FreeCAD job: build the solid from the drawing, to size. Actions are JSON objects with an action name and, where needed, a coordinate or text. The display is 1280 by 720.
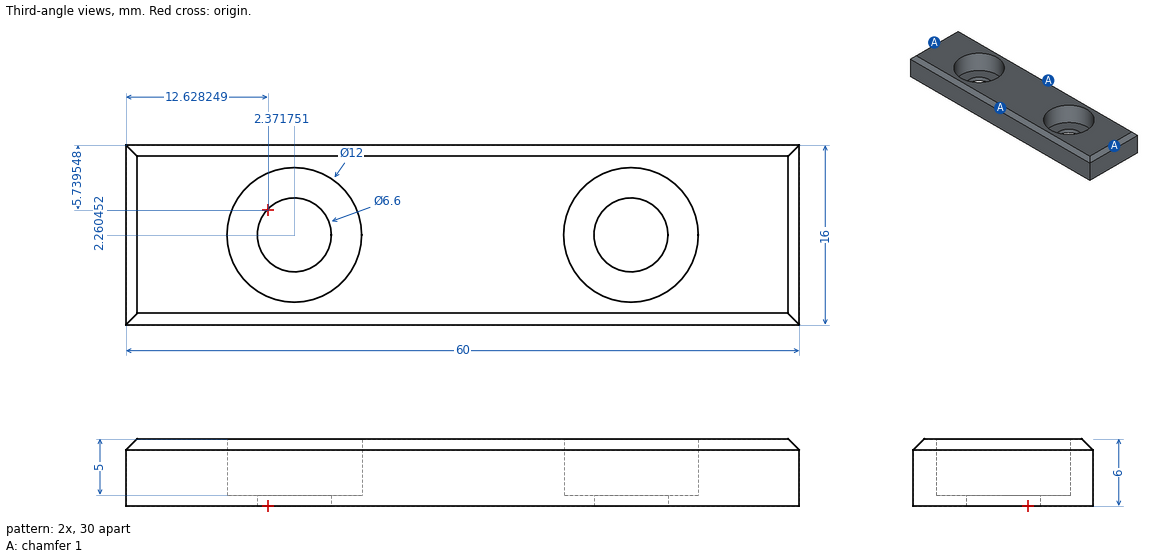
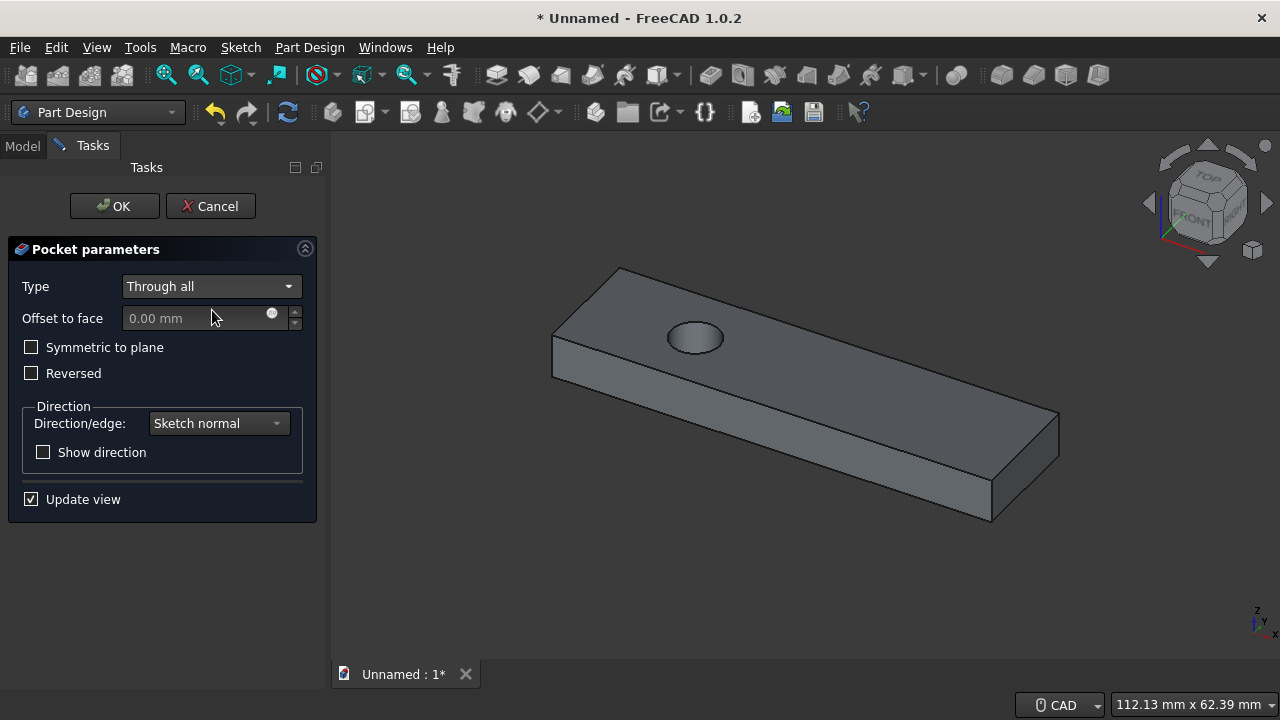
{"action": "left_click", "coordinate": [115, 206]}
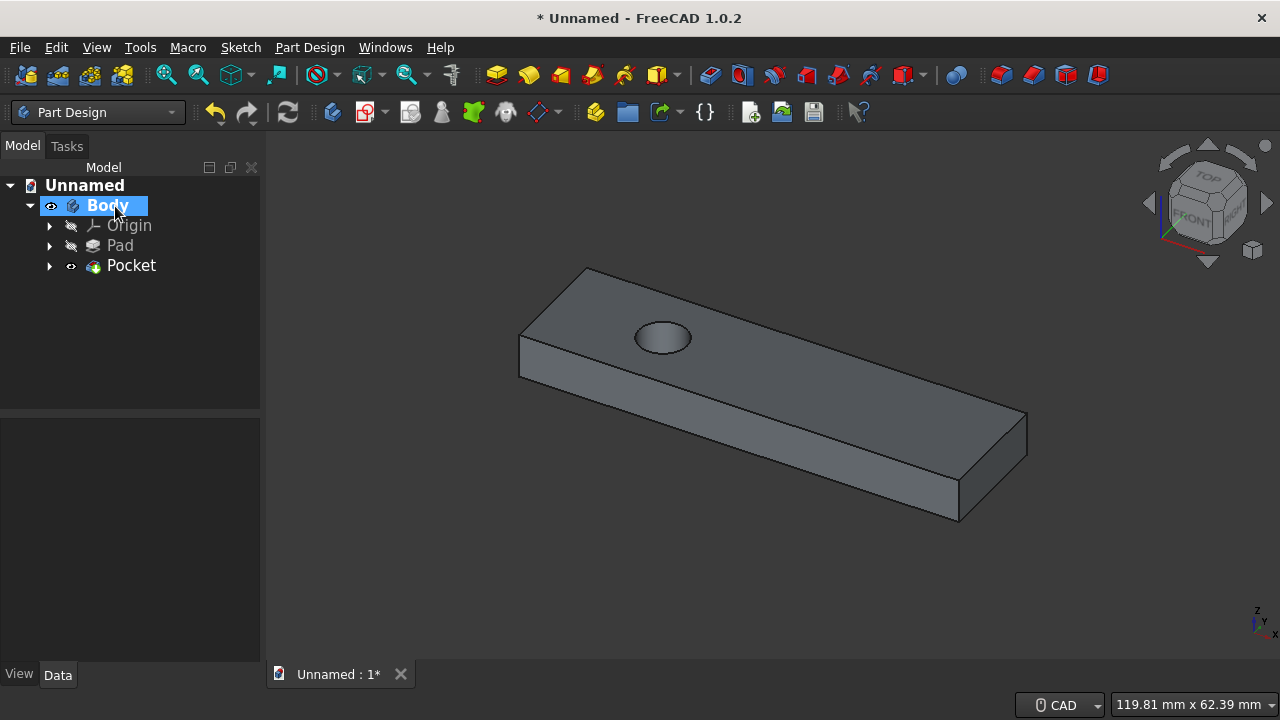
{"action": "left_click", "coordinate": [899, 415]}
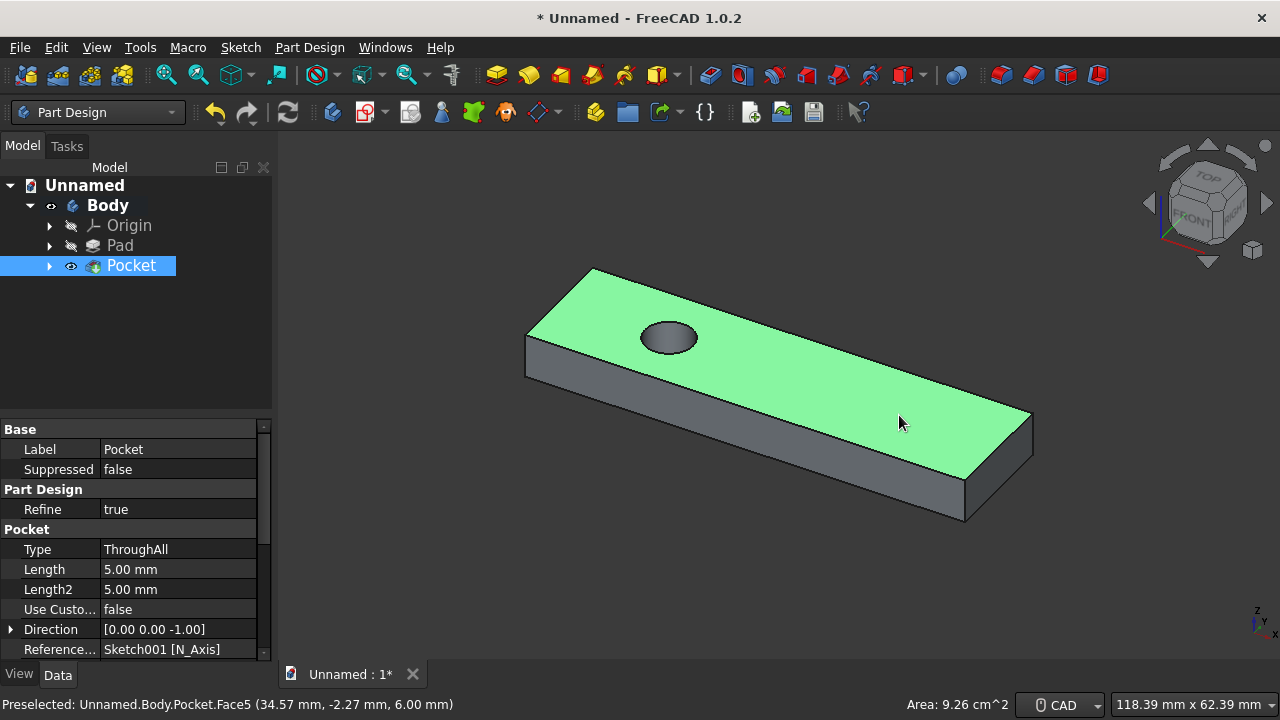
{"action": "left_click", "coordinate": [366, 112]}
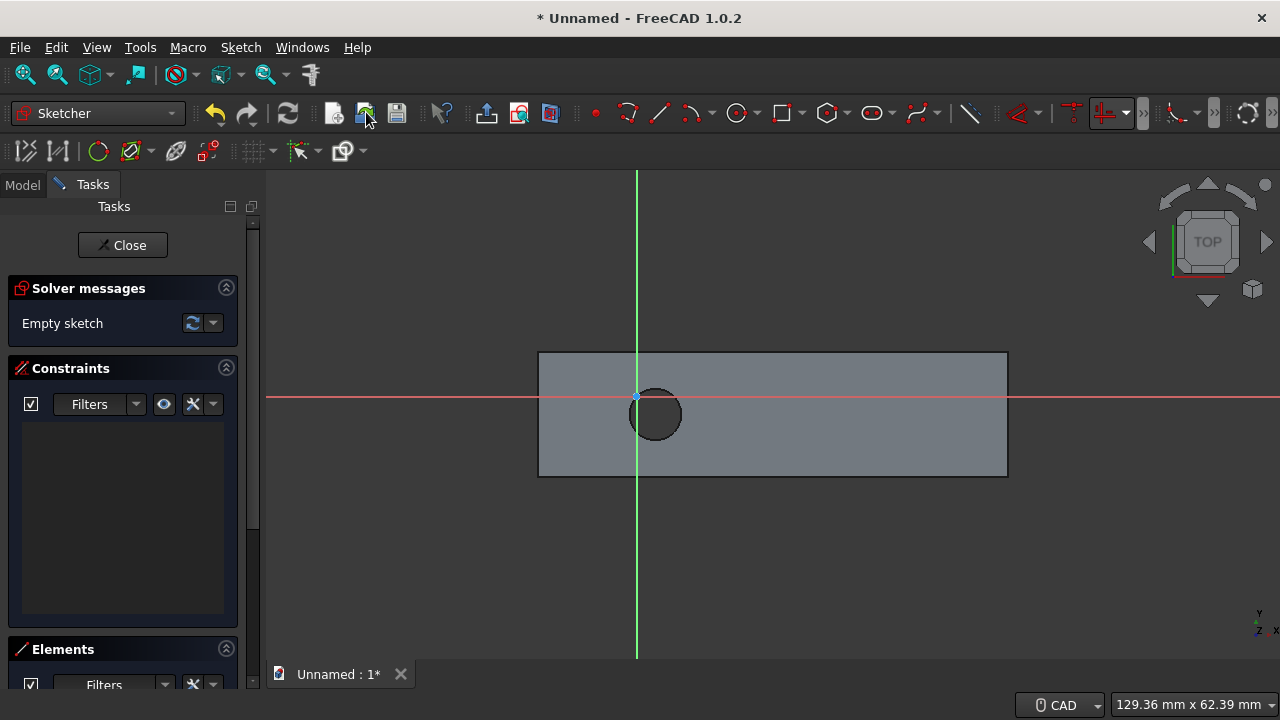
{"action": "scroll", "coordinate": [634, 415], "scroll_direction": "up", "scroll_amount": 6}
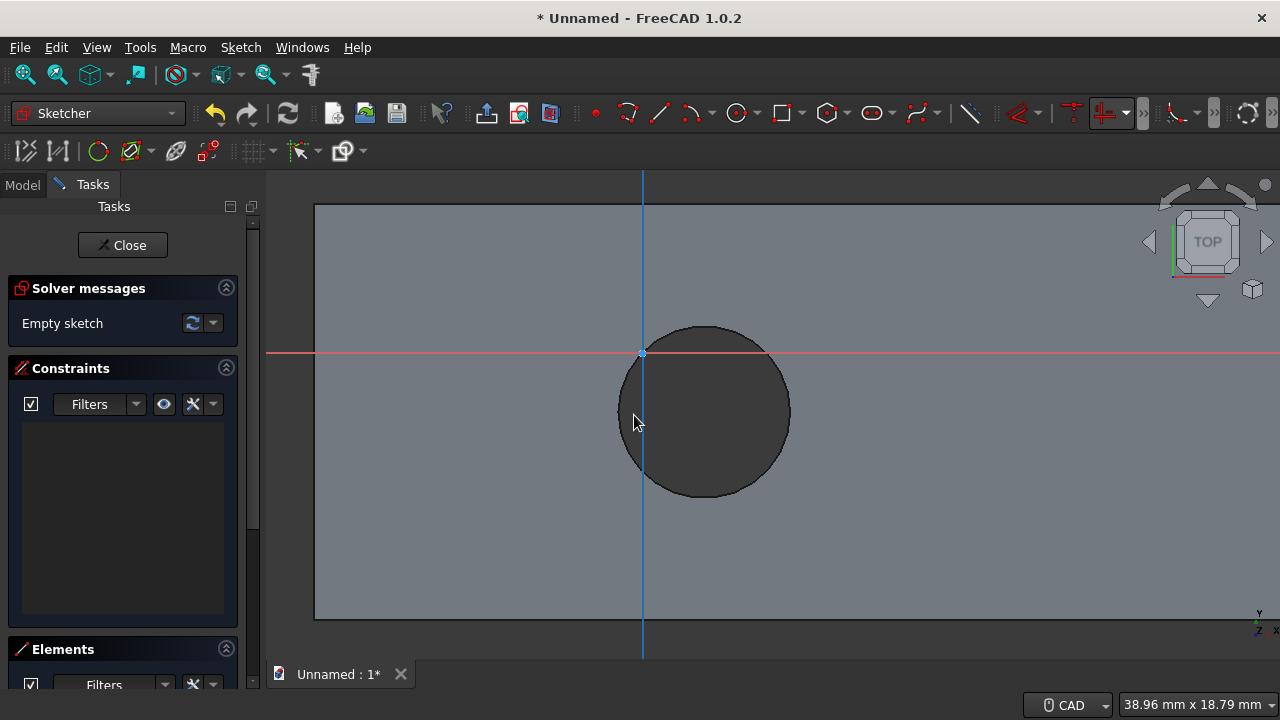
{"action": "left_click", "coordinate": [738, 114]}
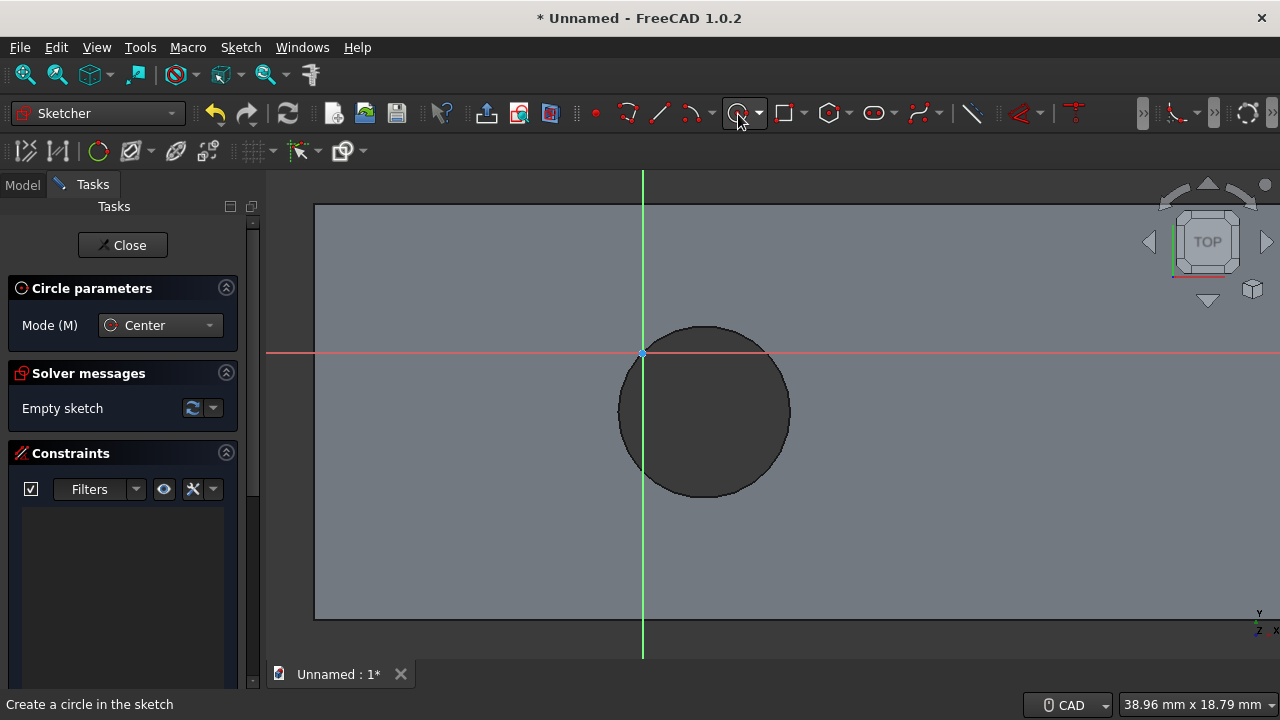
{"action": "left_click", "coordinate": [704, 412]}
{"action": "mouse_move", "coordinate": [815, 302]}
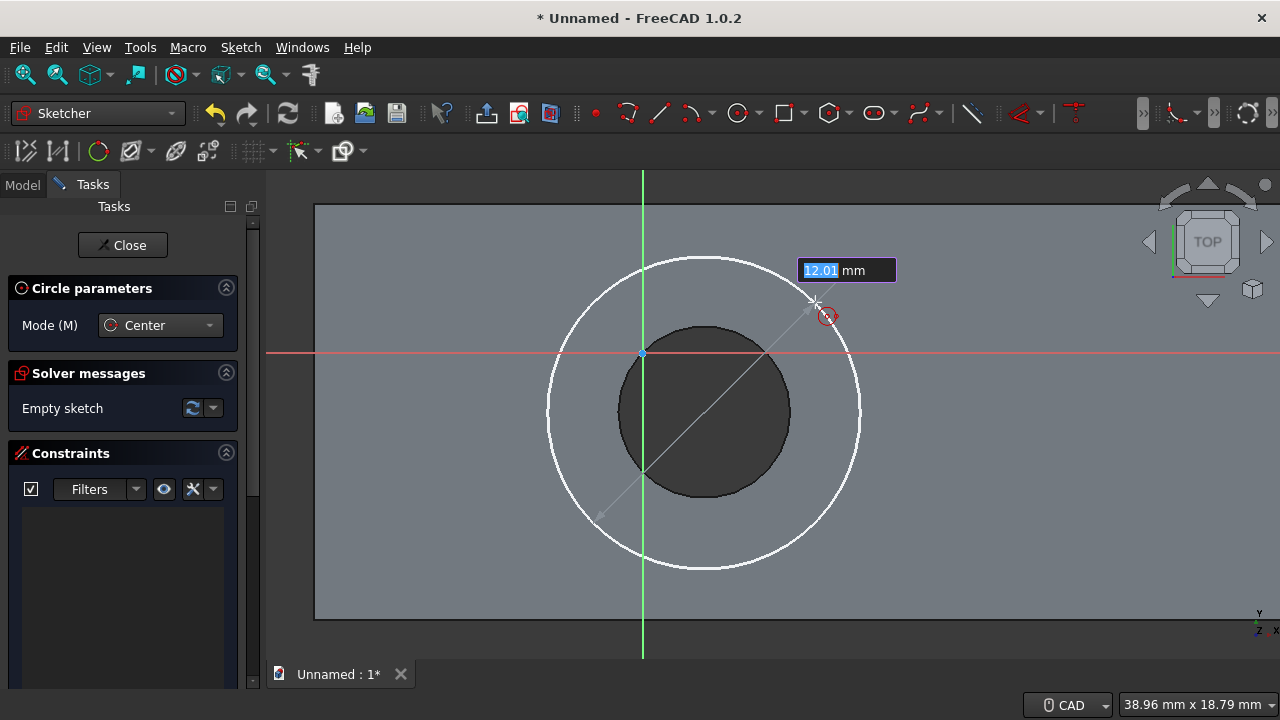
{"action": "type", "text": "12"}
{"action": "key", "text": "Return"}
{"action": "key", "text": "Escape"}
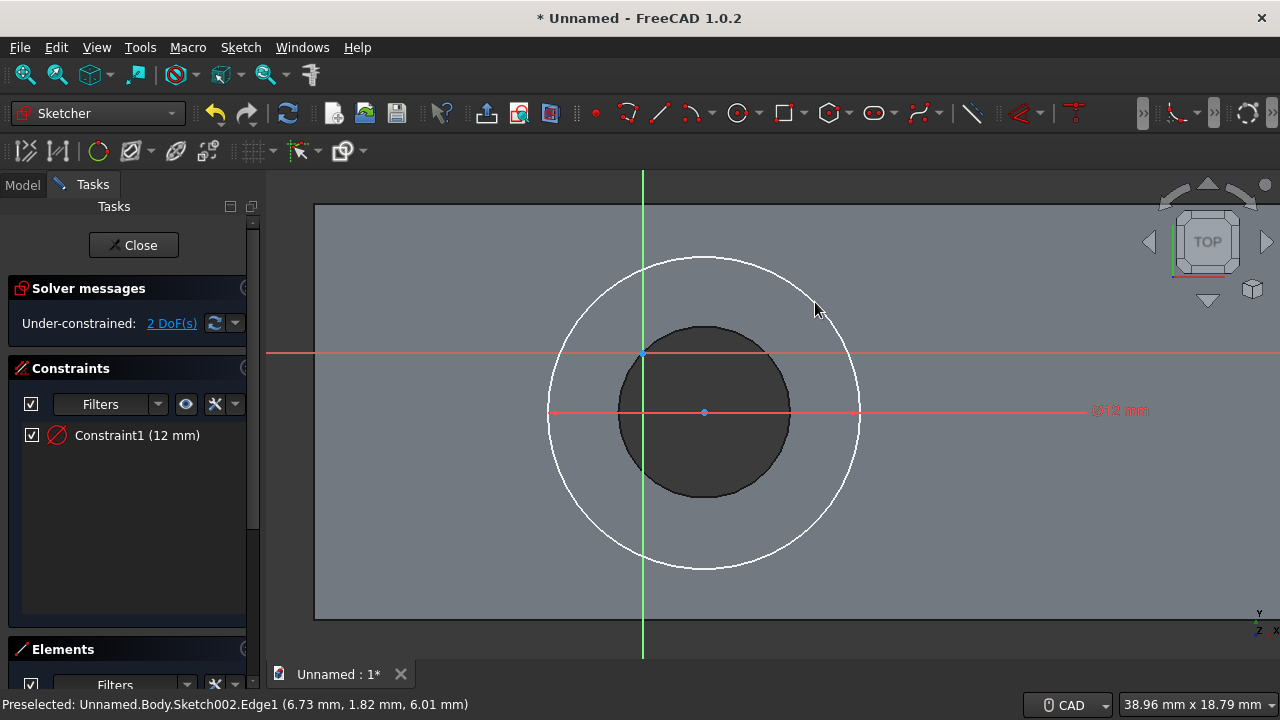
{"action": "left_click", "coordinate": [1020, 114]}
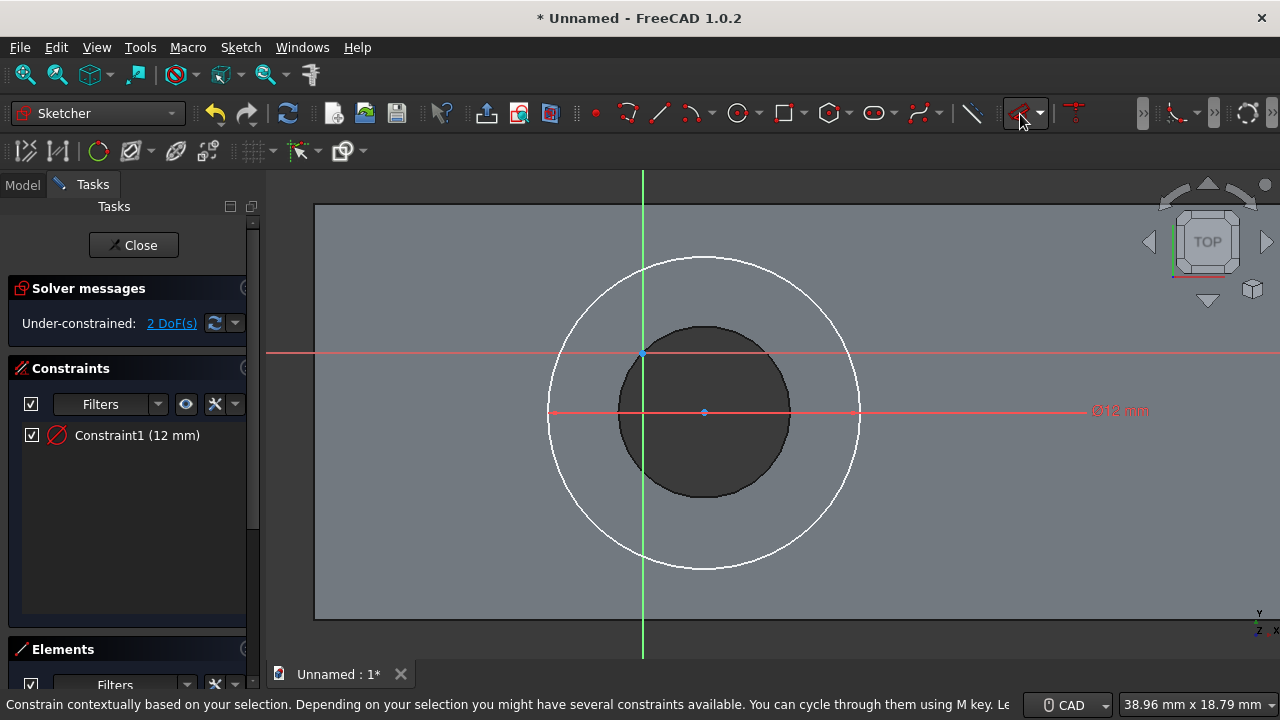
{"action": "left_click", "coordinate": [704, 413]}
{"action": "left_click", "coordinate": [673, 319]}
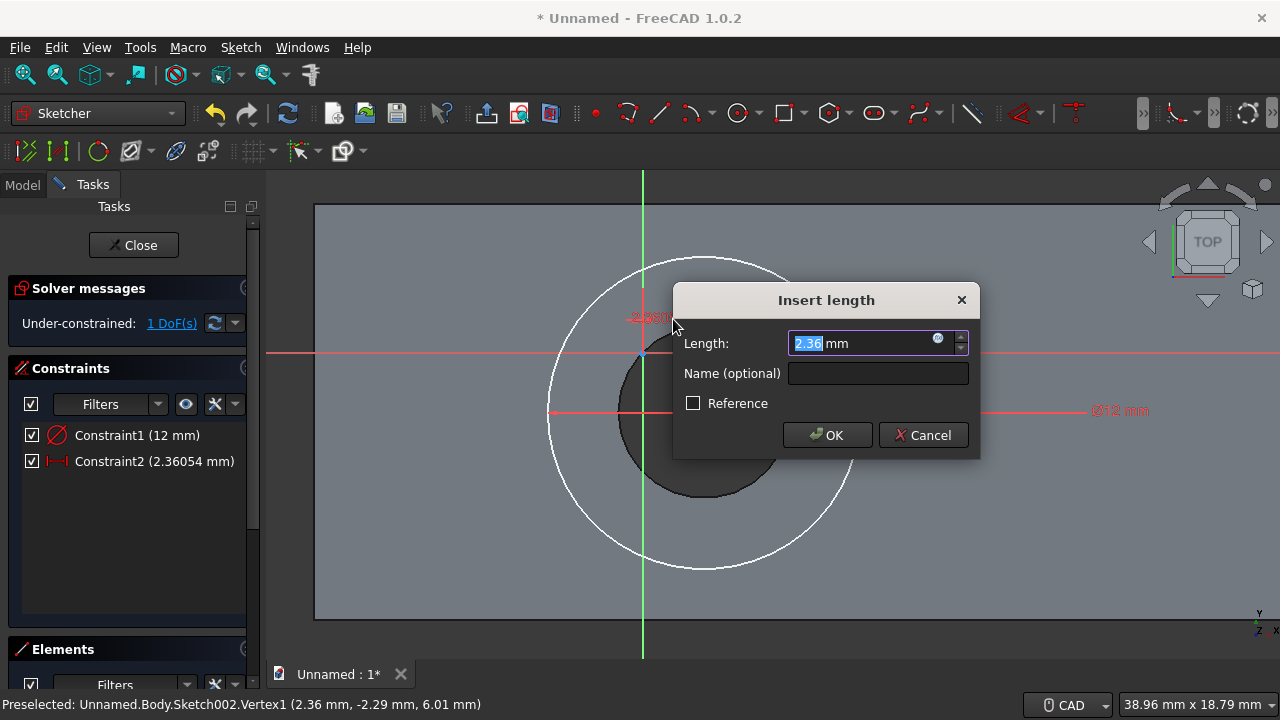
{"action": "type", "text": "2.371751"}
{"action": "key", "text": "Return"}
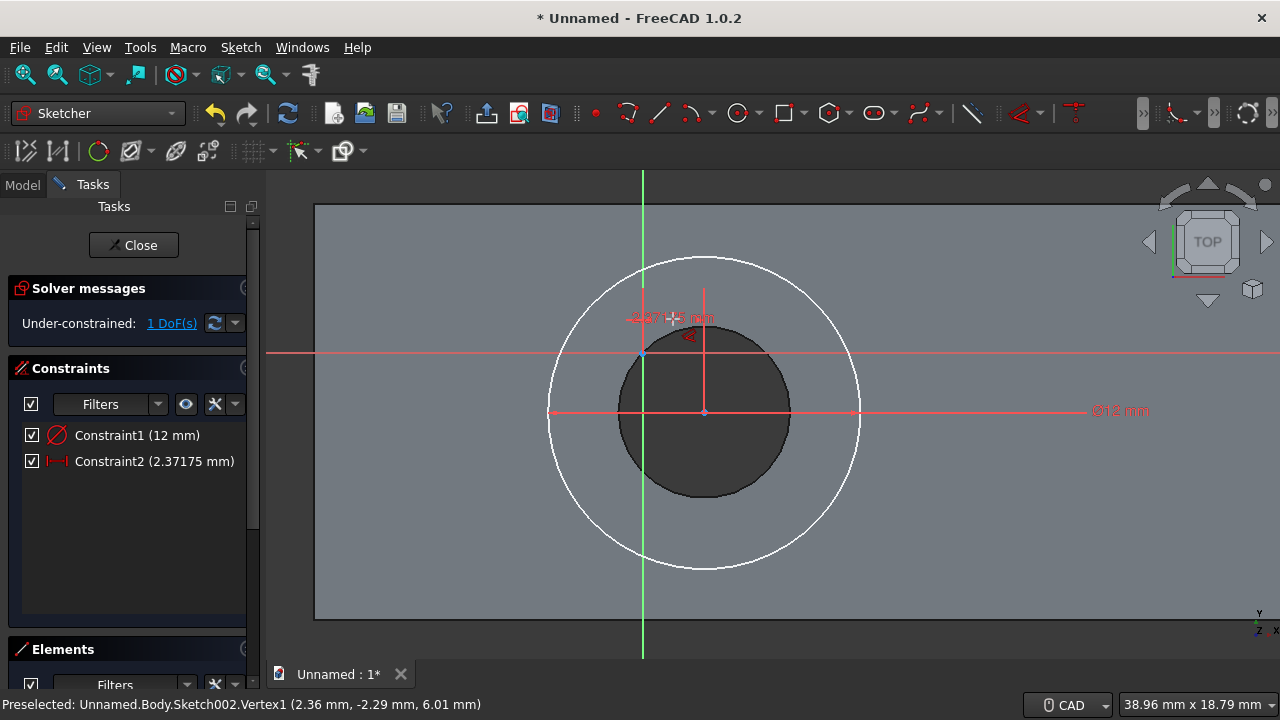
{"action": "left_click", "coordinate": [704, 413]}
{"action": "left_click", "coordinate": [609, 383]}